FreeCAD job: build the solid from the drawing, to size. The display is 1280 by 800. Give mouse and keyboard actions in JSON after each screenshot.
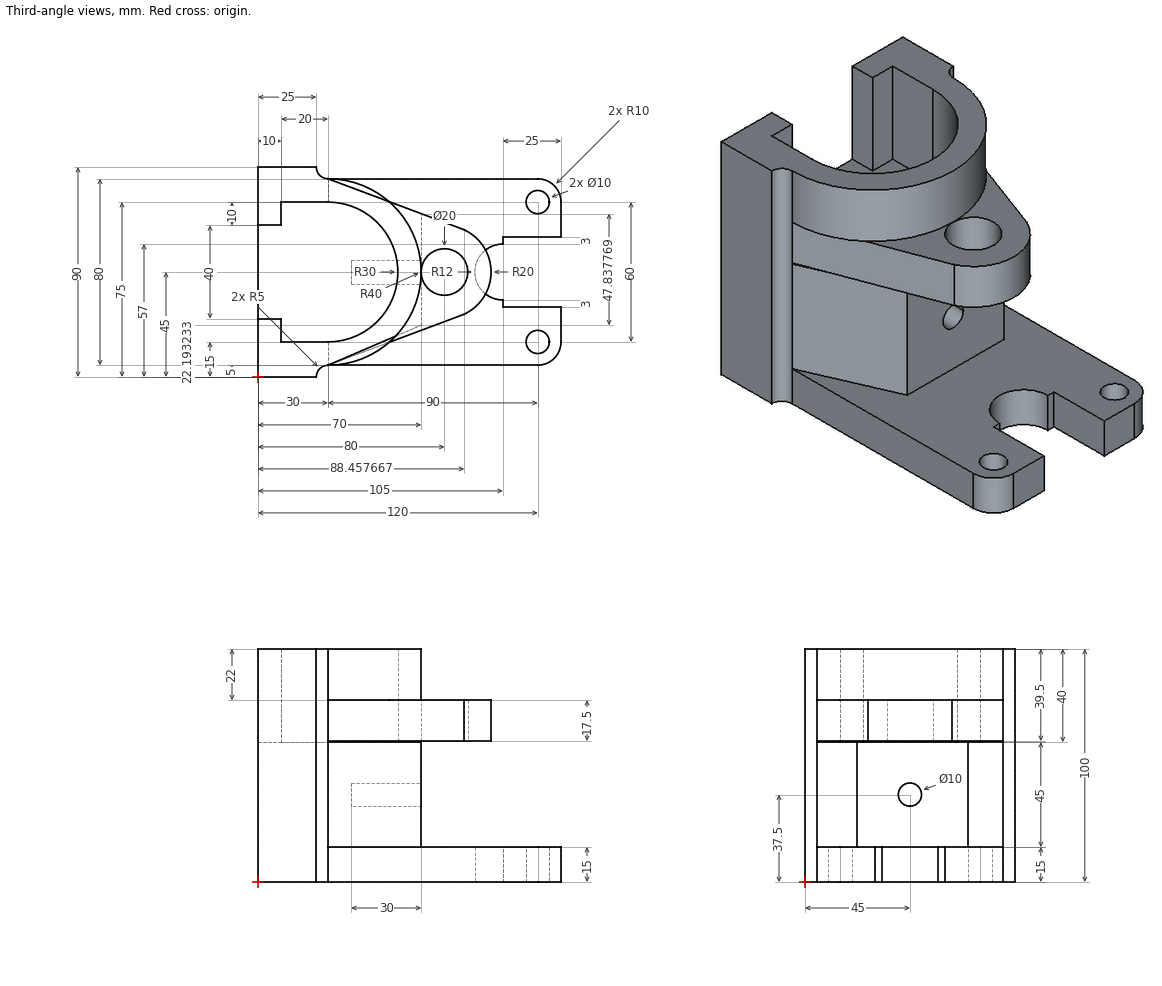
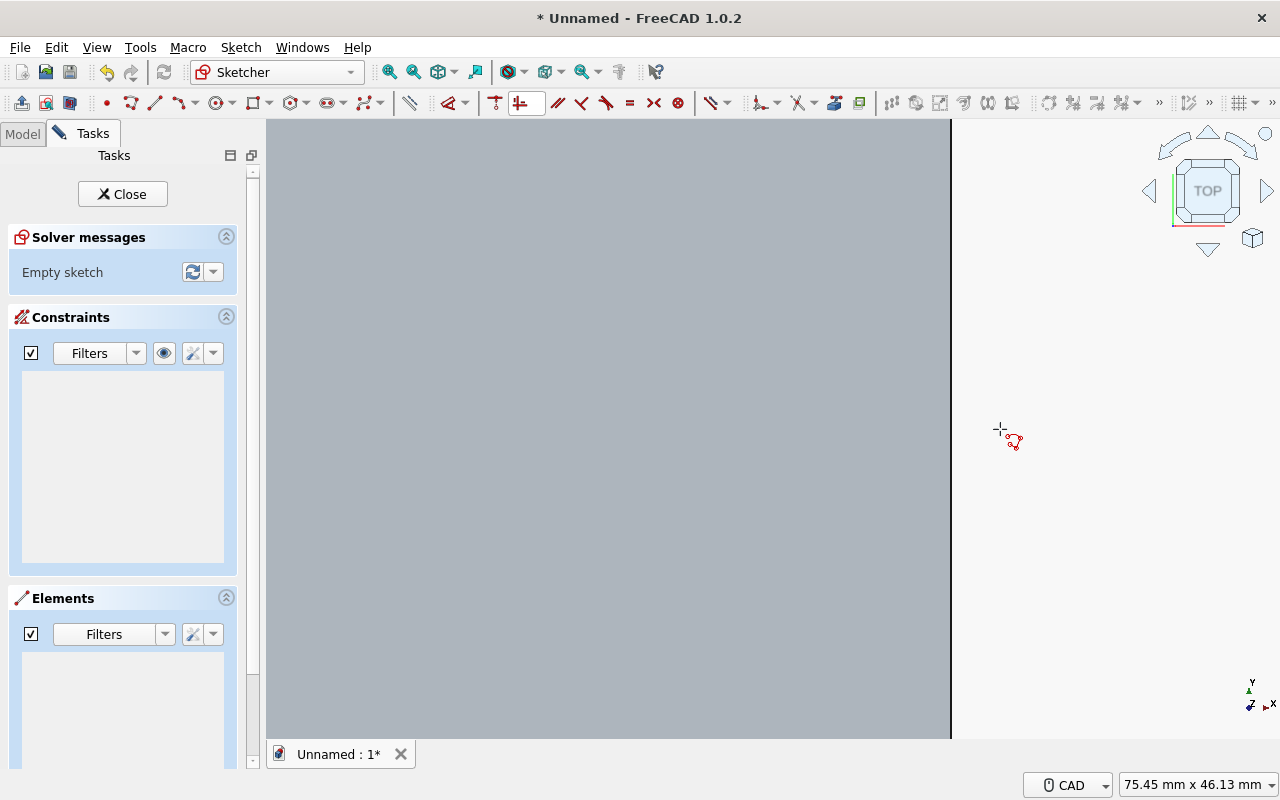
{"action": "left_click", "coordinate": [615, 266]}
{"action": "left_click", "coordinate": [615, 226]}
{"action": "left_click", "coordinate": [951, 226]}
{"action": "left_click", "coordinate": [951, 629]}
{"action": "left_click", "coordinate": [615, 629]}
{"action": "left_click", "coordinate": [615, 589]}
{"action": "right_click", "coordinate": [615, 589]}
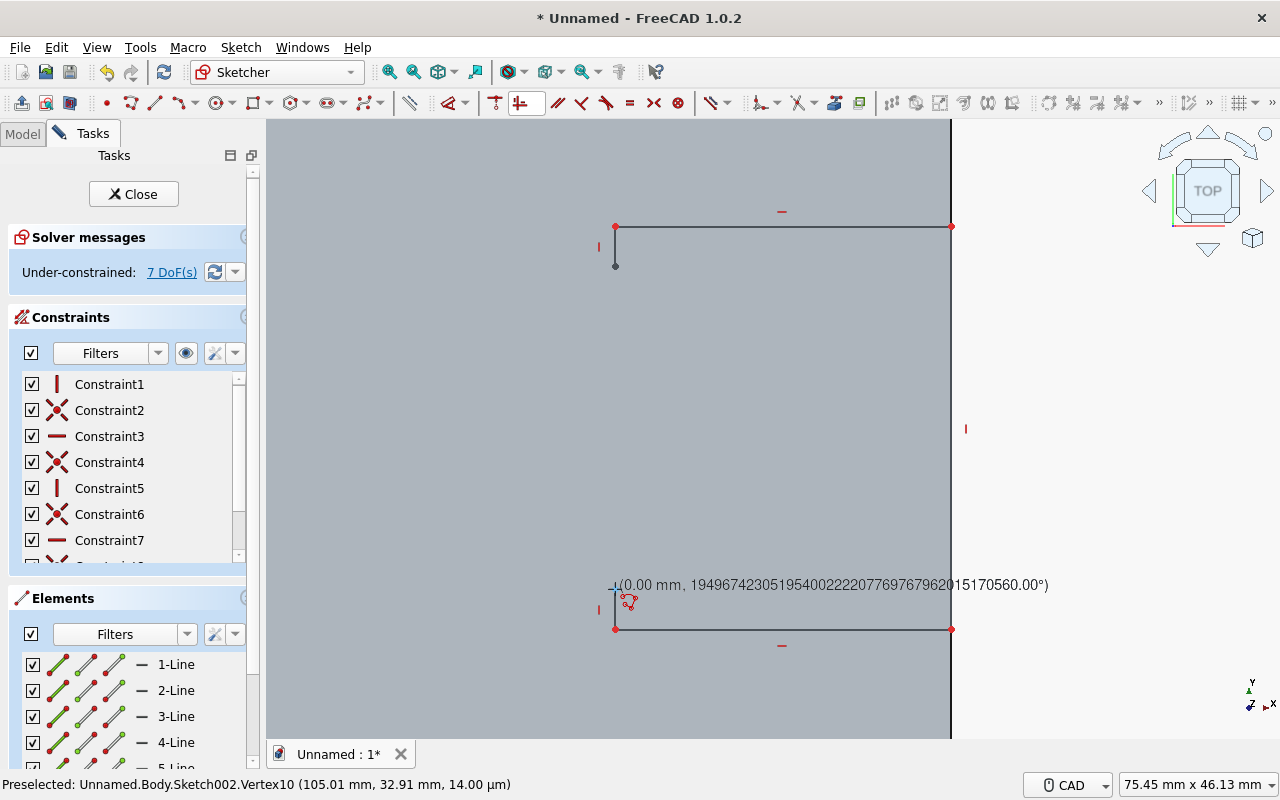
{"action": "left_click", "coordinate": [180, 104]}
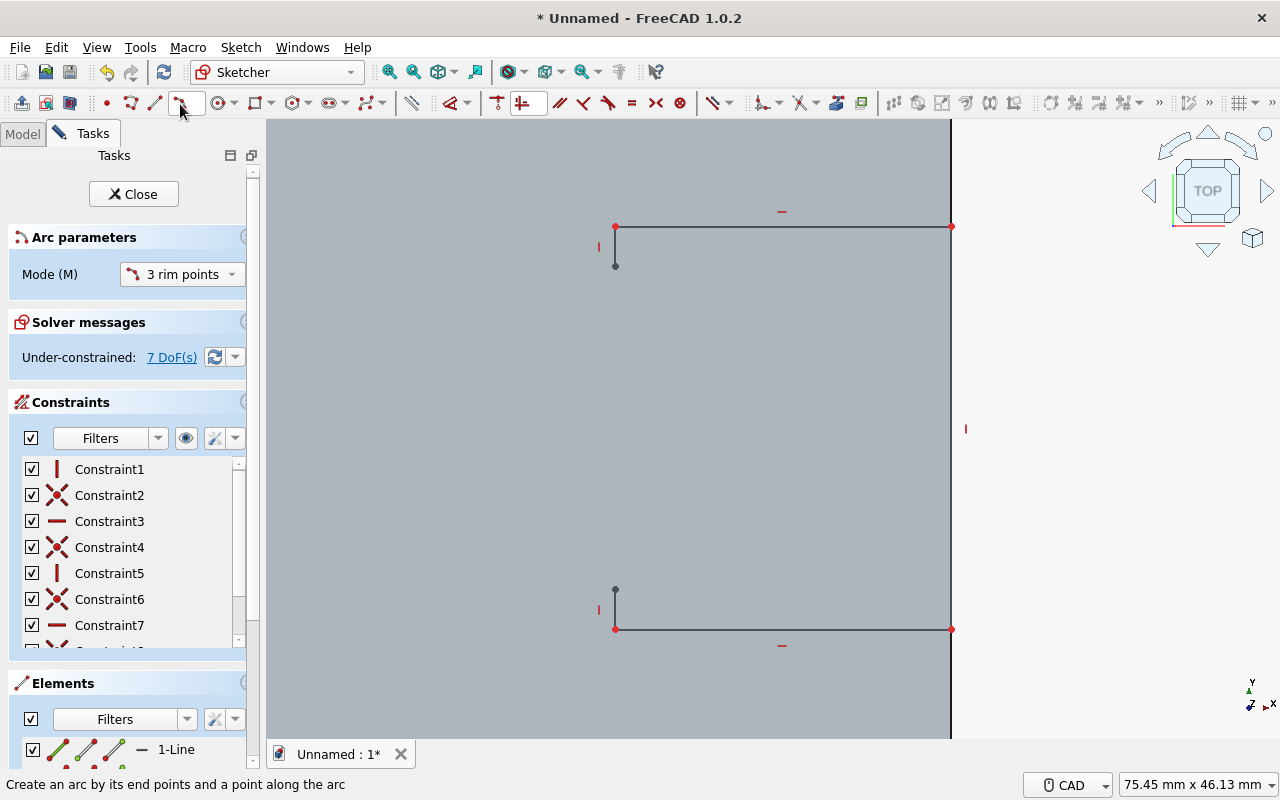
{"action": "left_click", "coordinate": [615, 590]}
{"action": "left_click", "coordinate": [615, 267]}
{"action": "left_click", "coordinate": [454, 427]}
{"action": "key", "text": "Escape"}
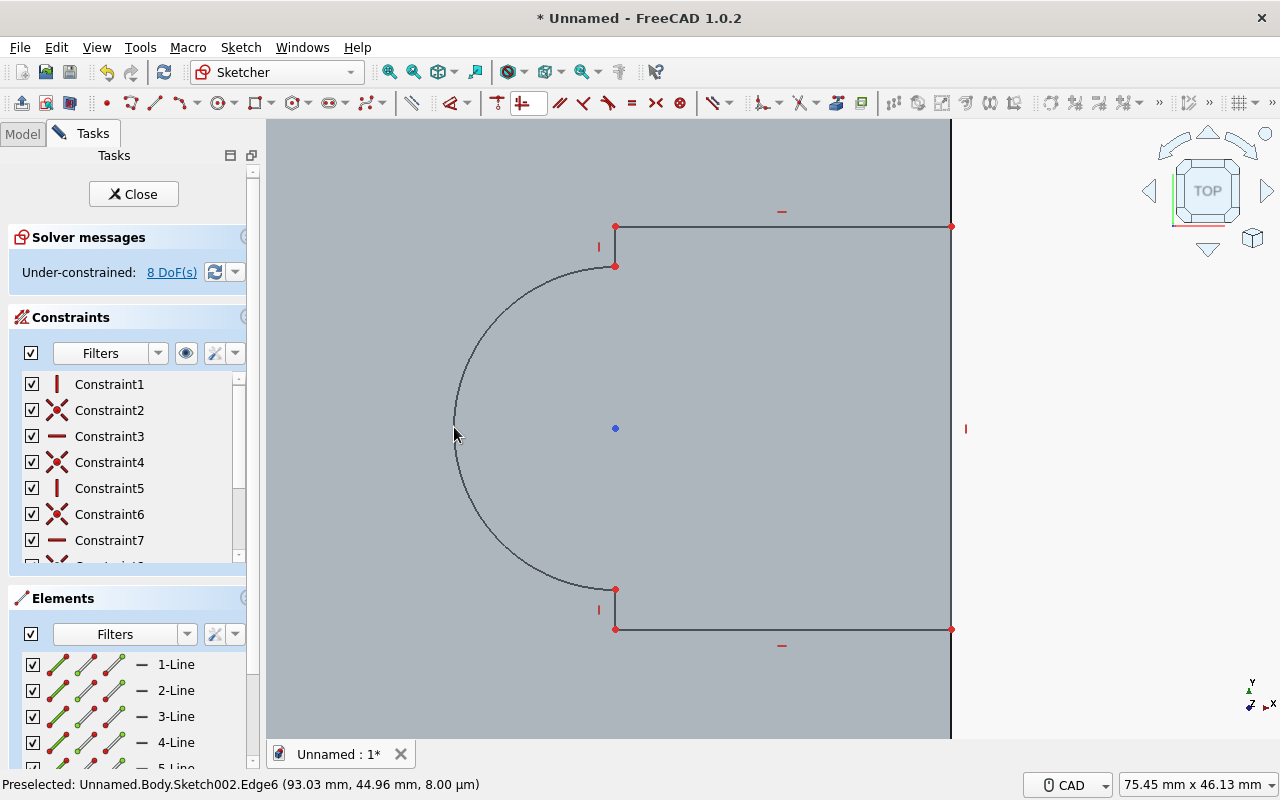
{"action": "left_click", "coordinate": [450, 104]}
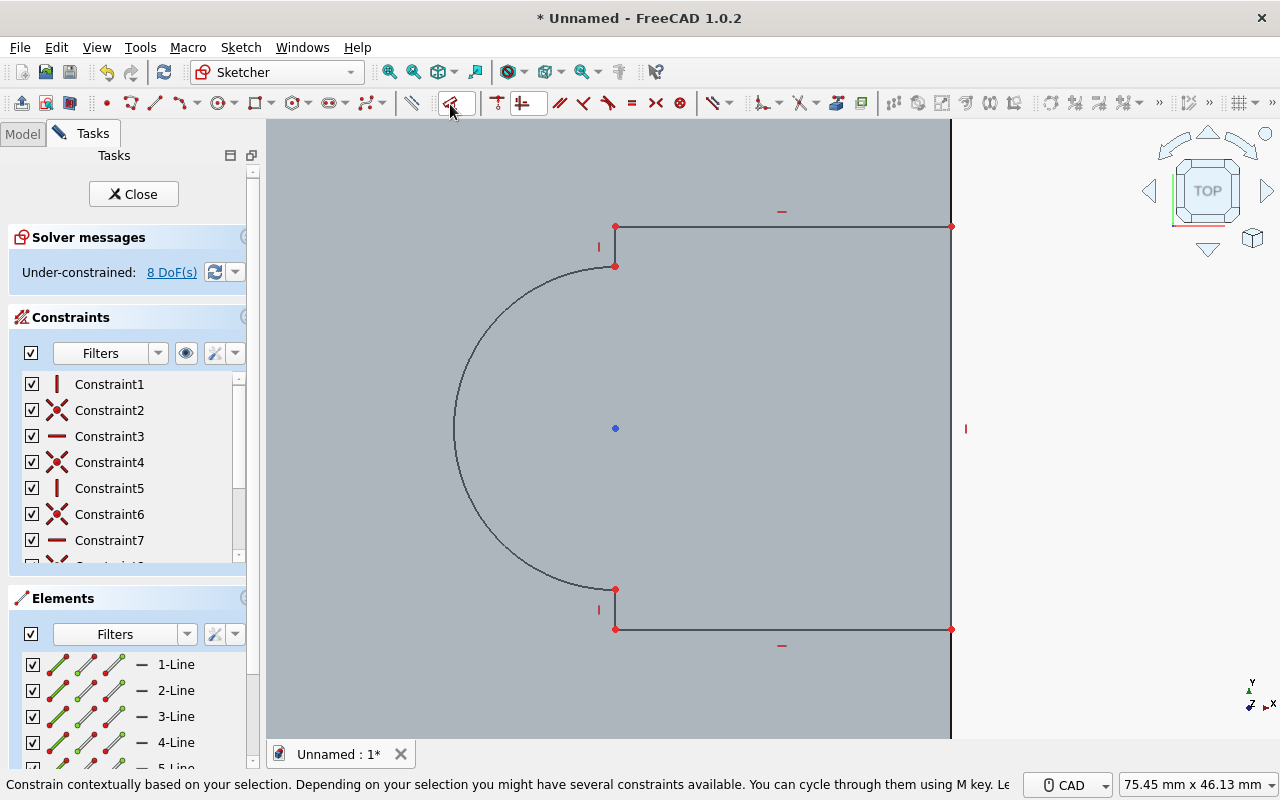
{"action": "left_click", "coordinate": [485, 334]}
{"action": "left_click", "coordinate": [459, 315]}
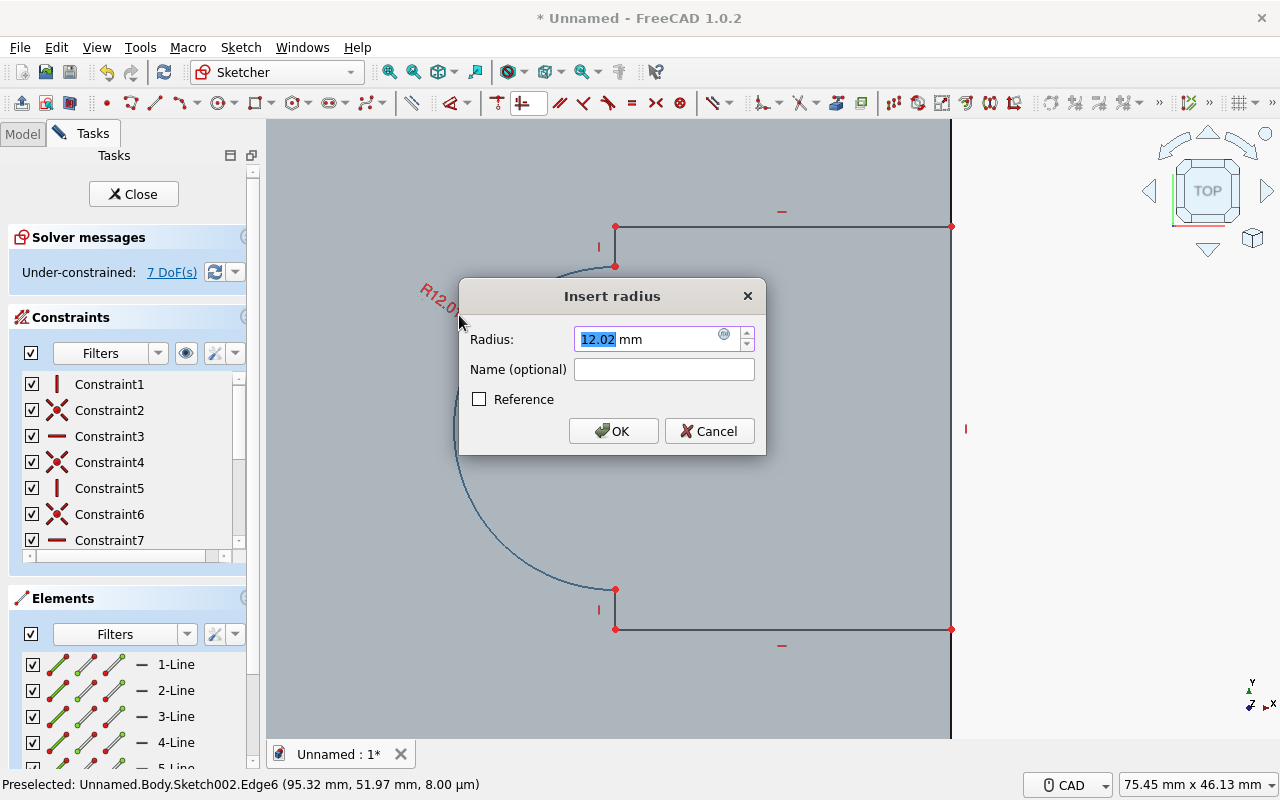
{"action": "type", "text": "12"}
{"action": "key", "text": "Return"}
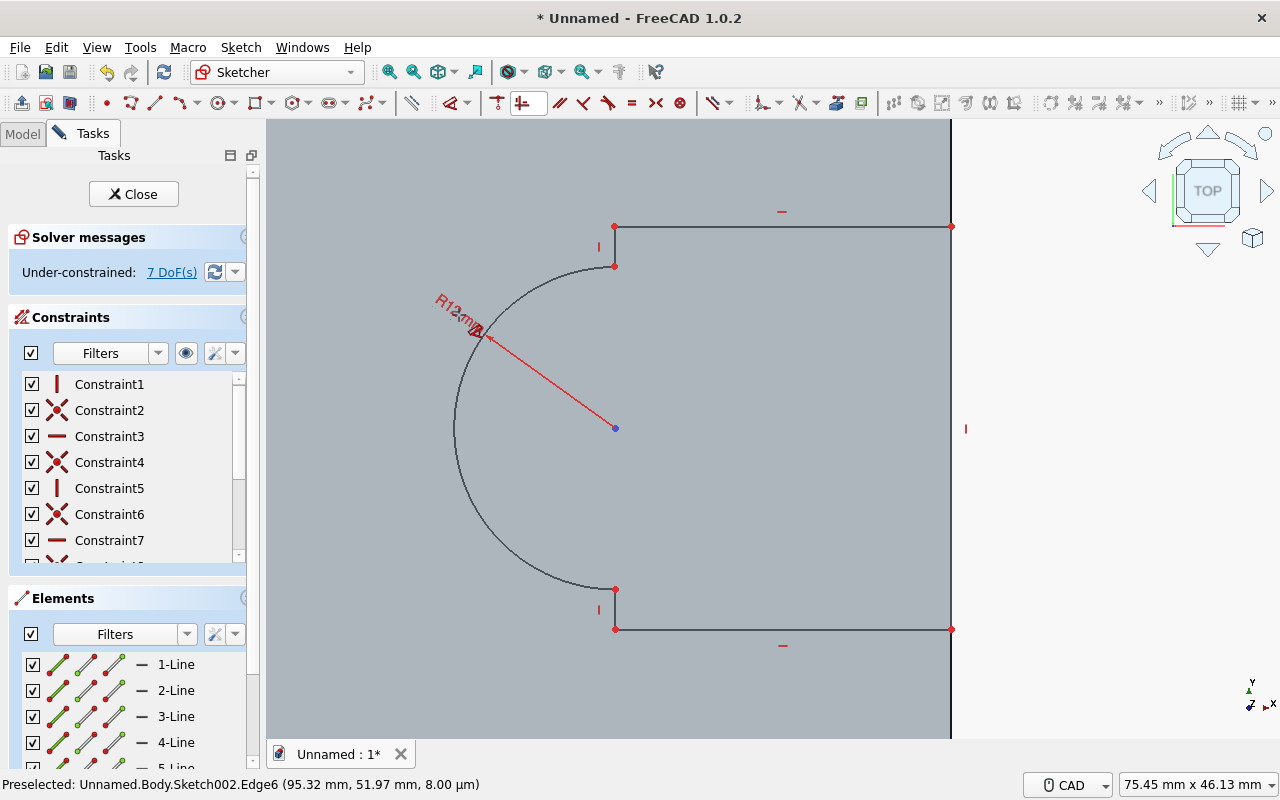
{"action": "left_click", "coordinate": [615, 255]}
{"action": "left_click", "coordinate": [581, 247]}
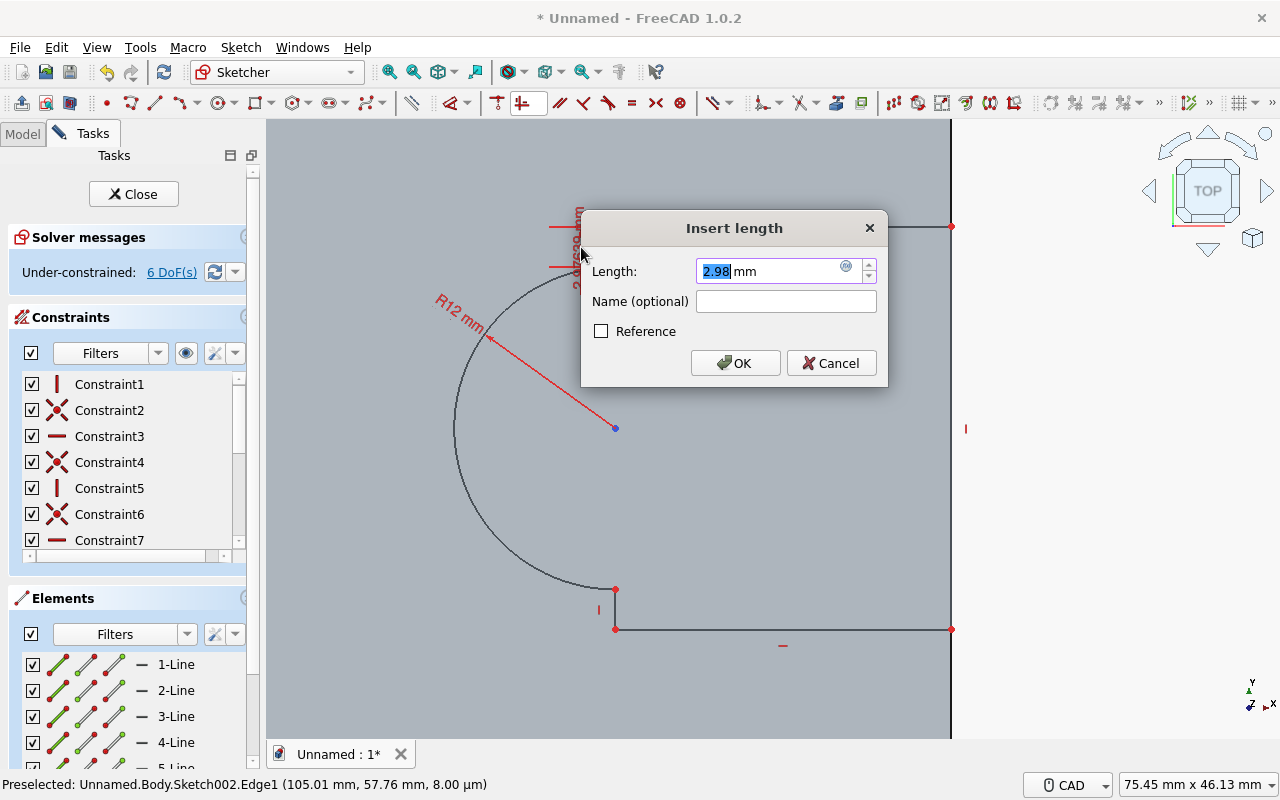
{"action": "type", "text": "3"}
{"action": "key", "text": "Return"}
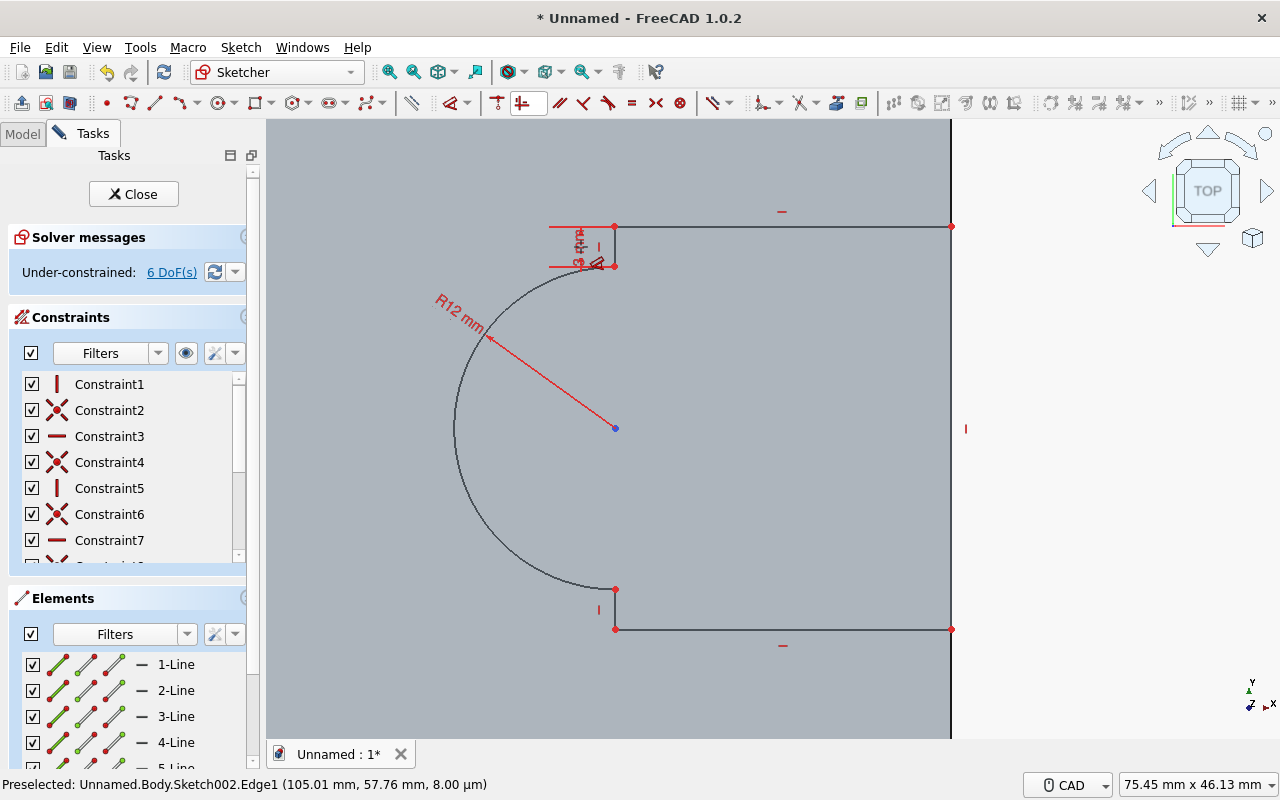
{"action": "left_click", "coordinate": [615, 618]}
{"action": "left_click", "coordinate": [581, 610]}